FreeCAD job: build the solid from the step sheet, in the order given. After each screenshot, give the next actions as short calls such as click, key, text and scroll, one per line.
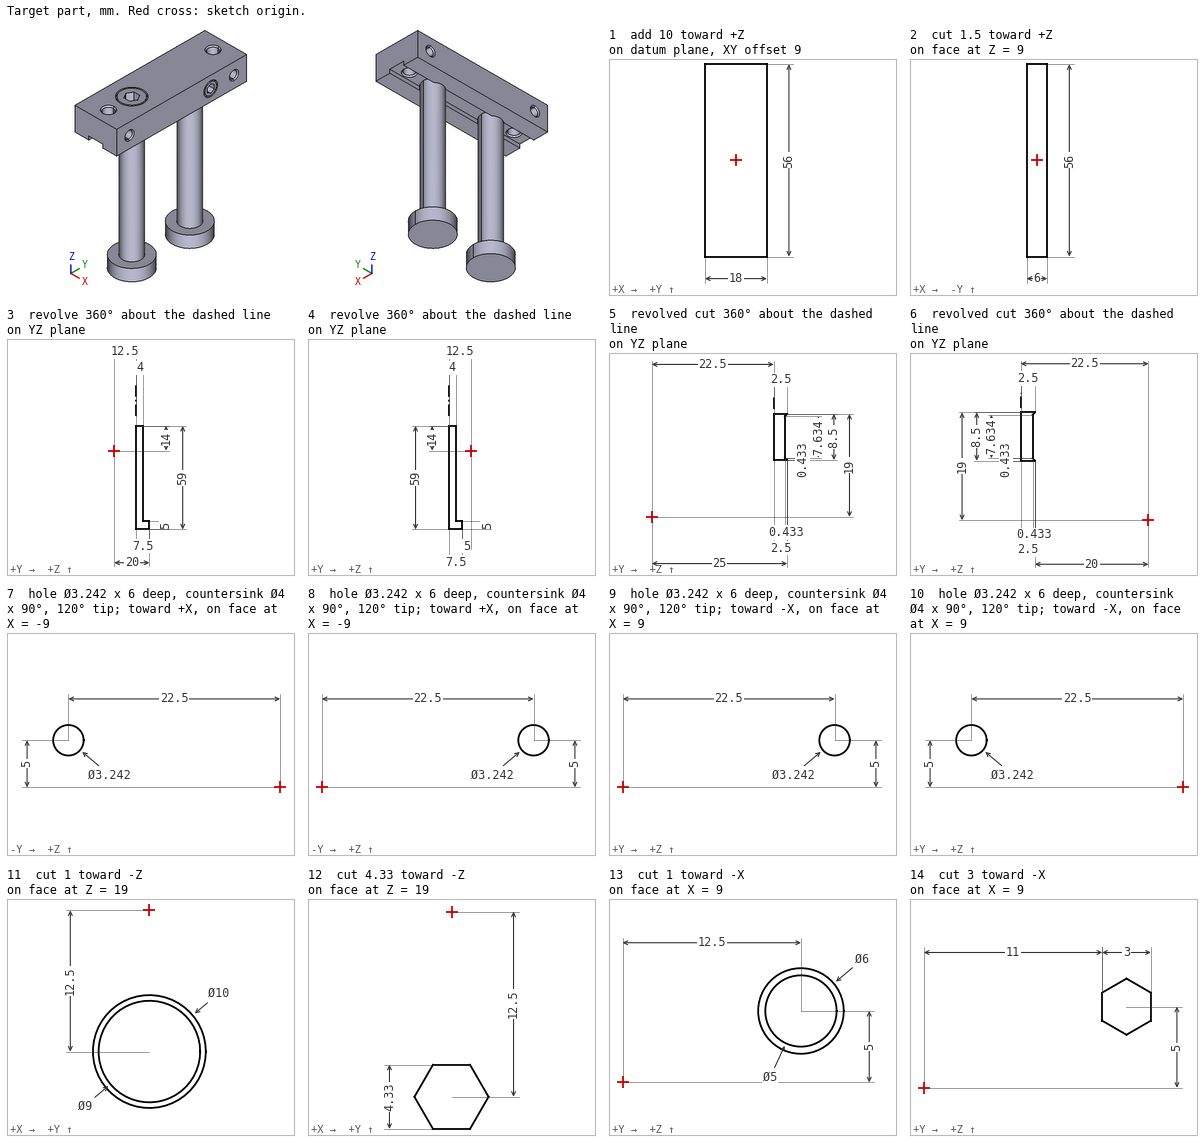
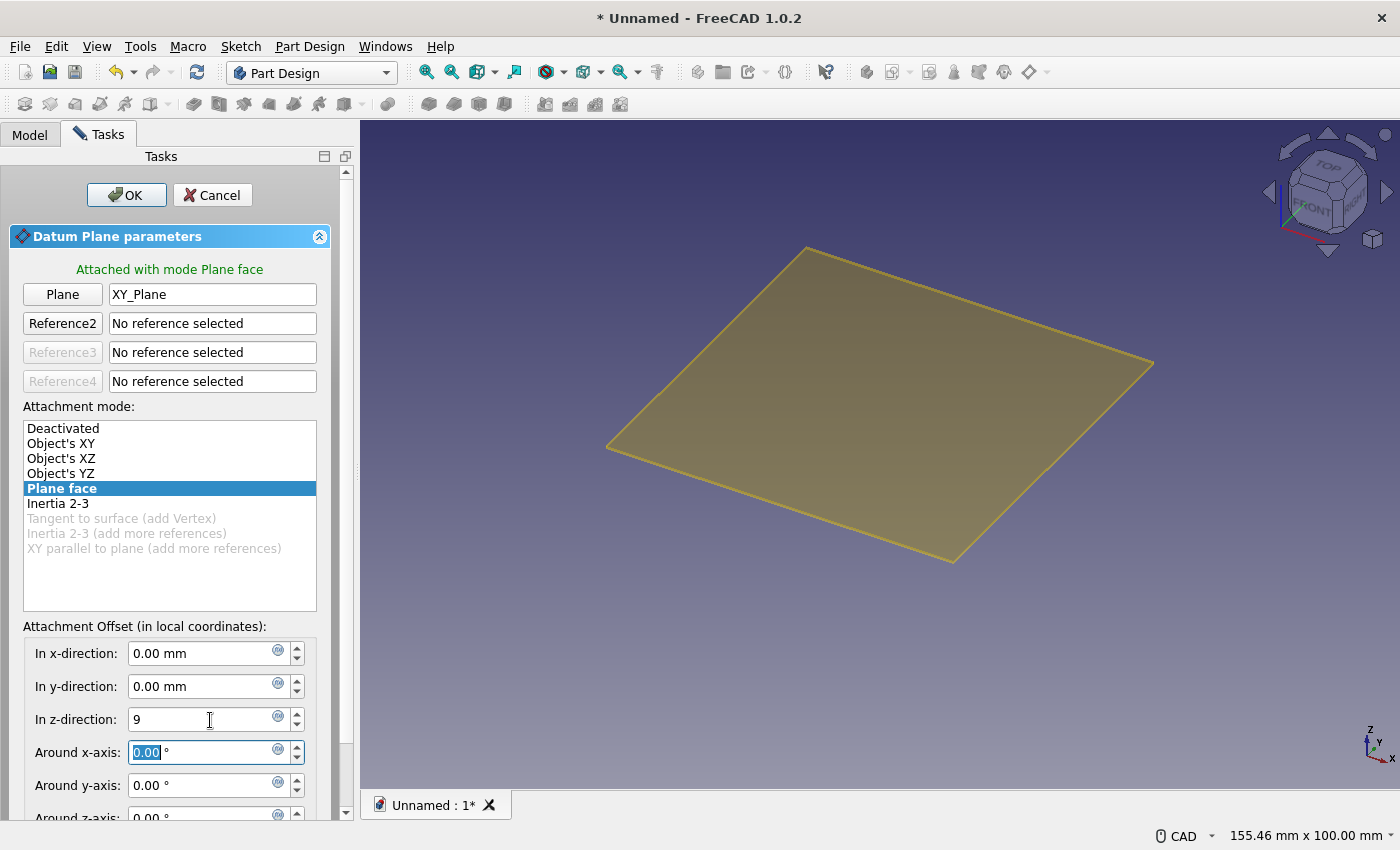
click(127, 195)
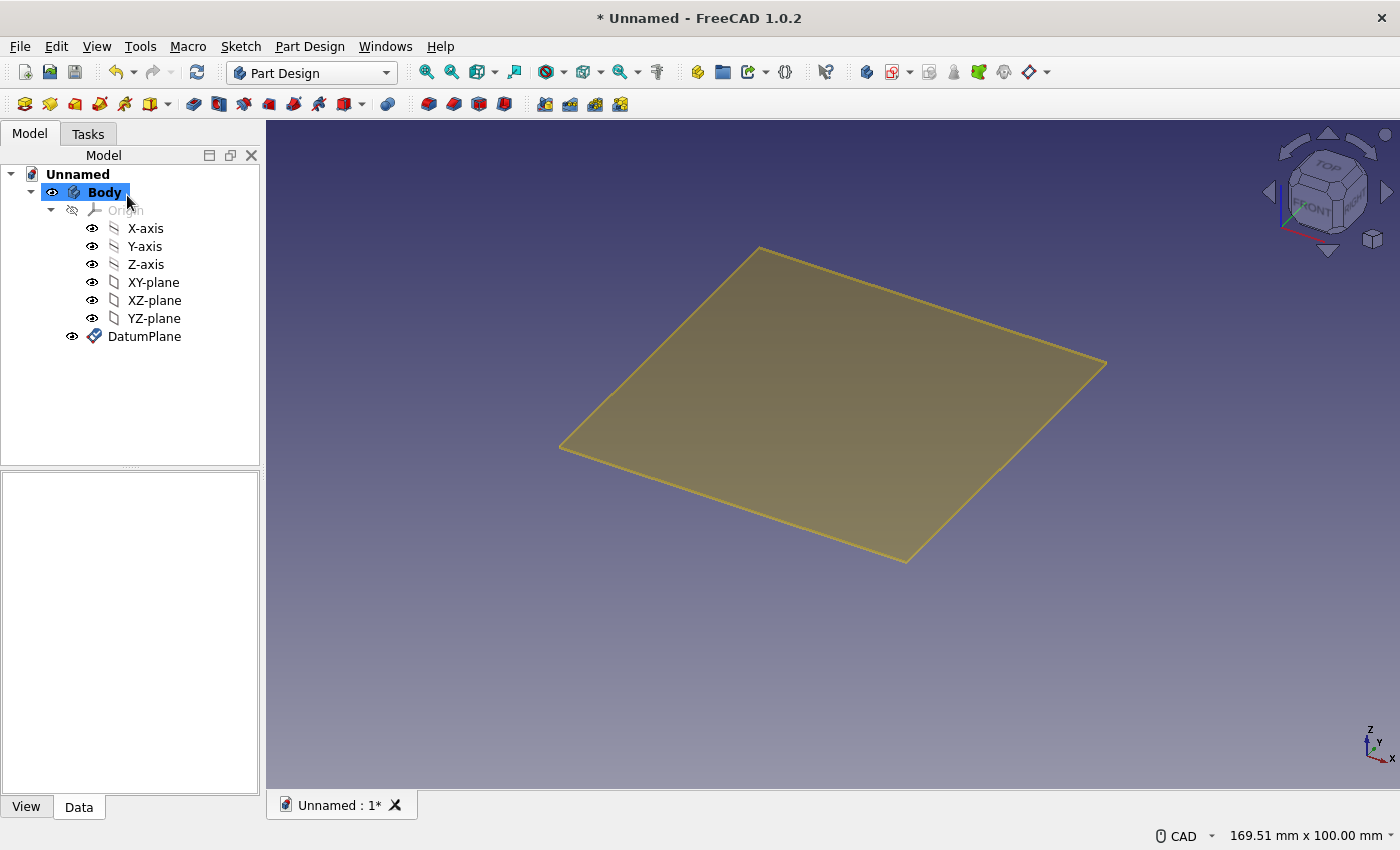
click(117, 336)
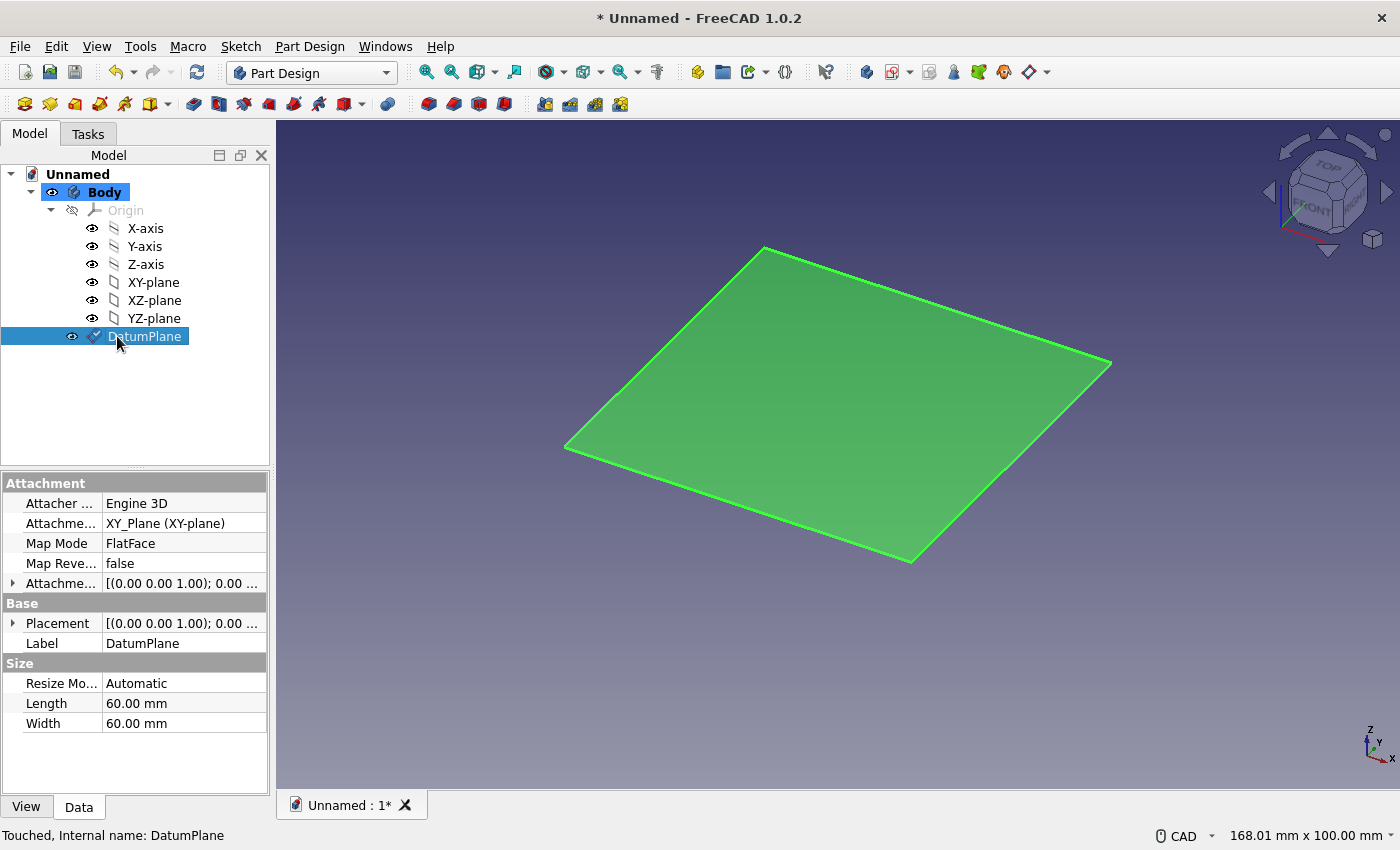
click(892, 72)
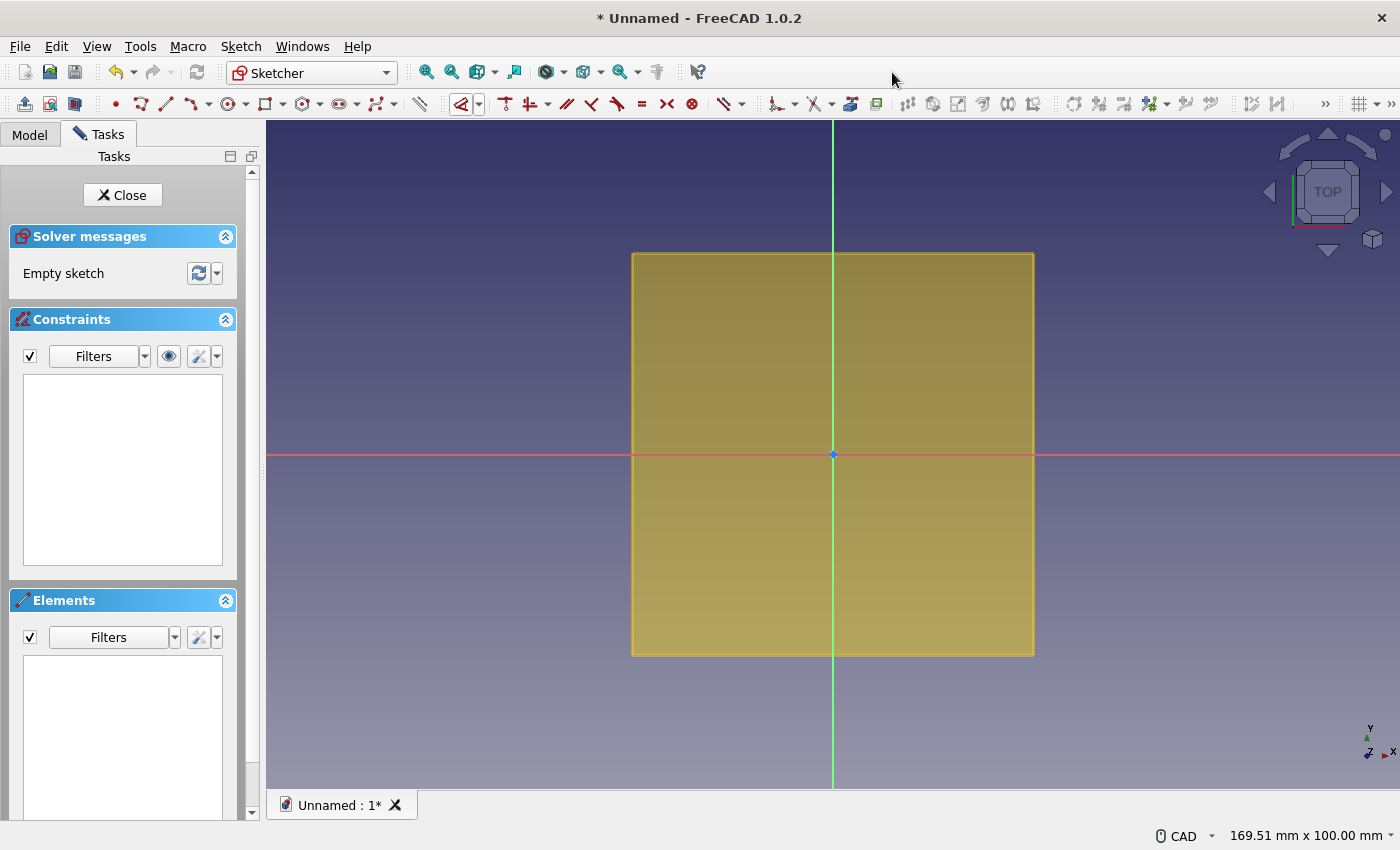
click(282, 104)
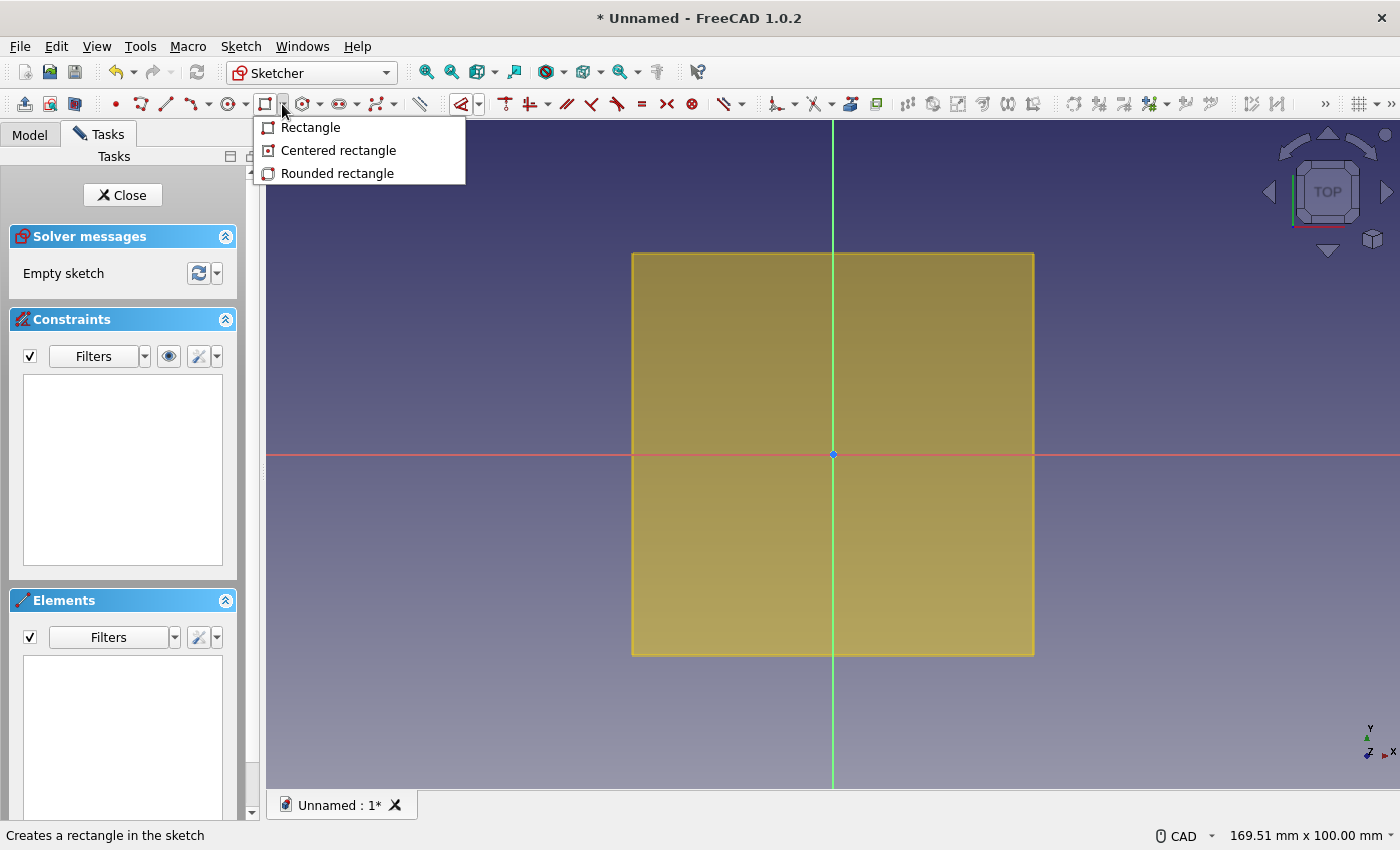
click(360, 150)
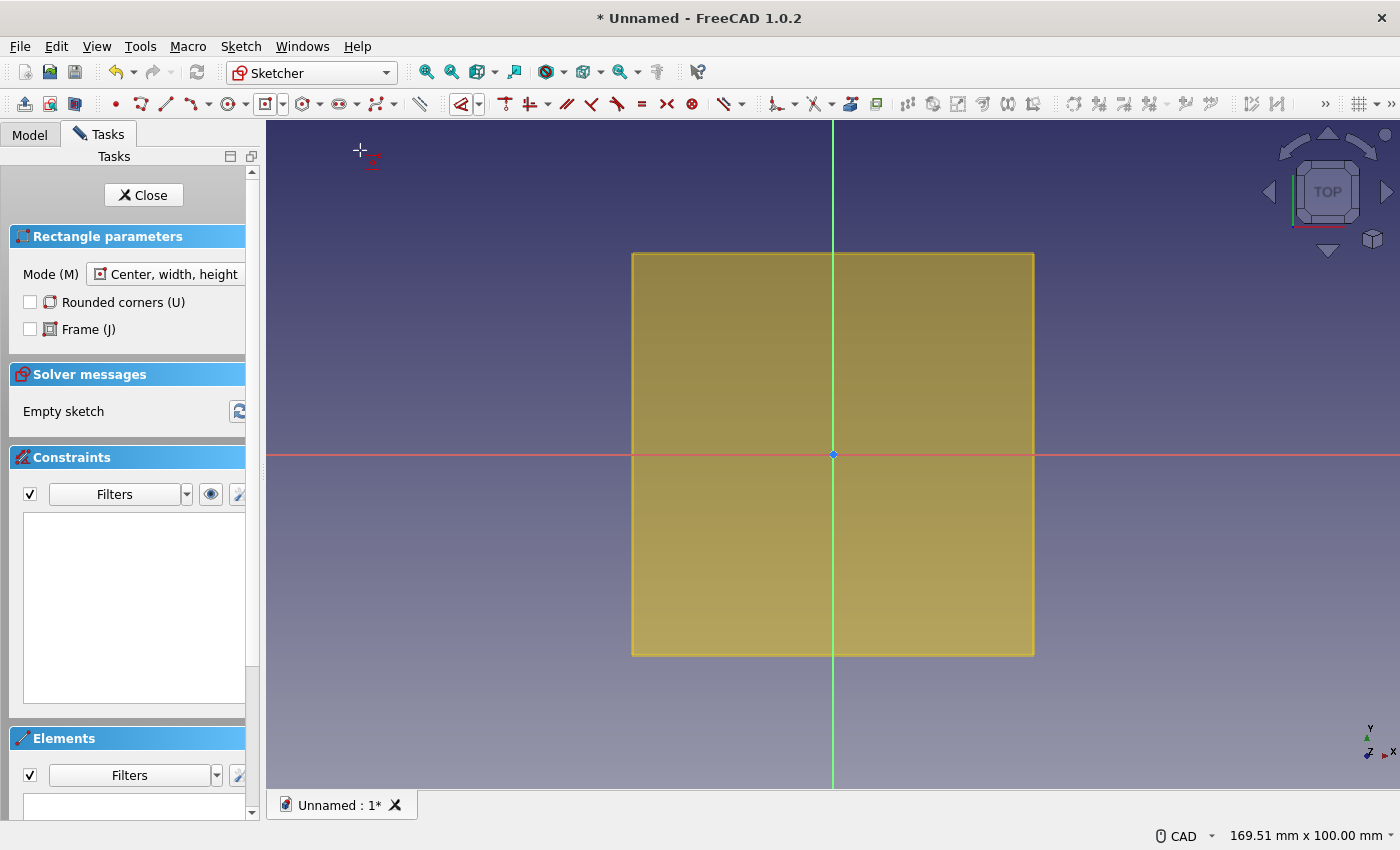
click(833, 454)
move(893, 267)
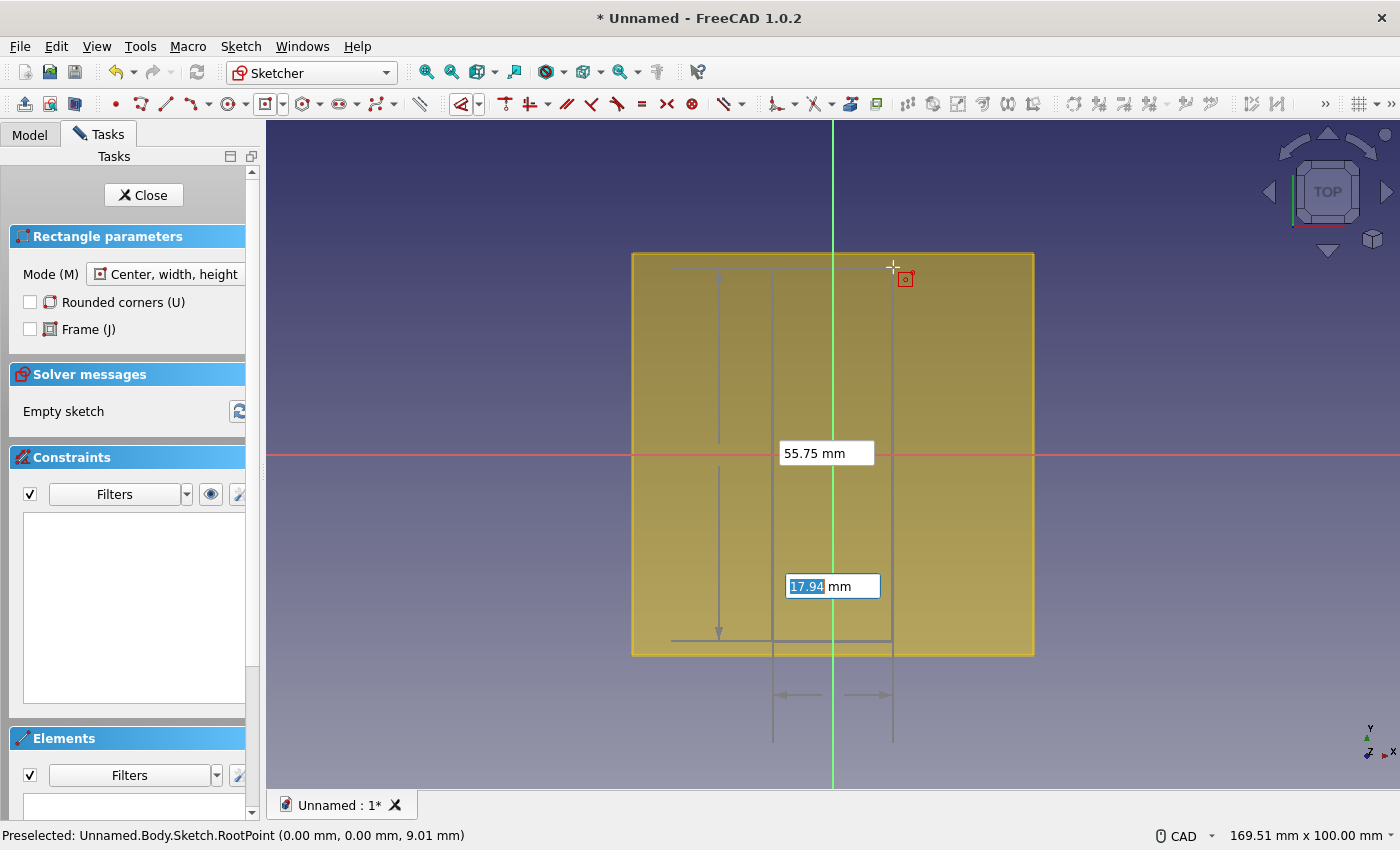
text(18)
key(Tab)
text(56)
key(Return)
key(Escape)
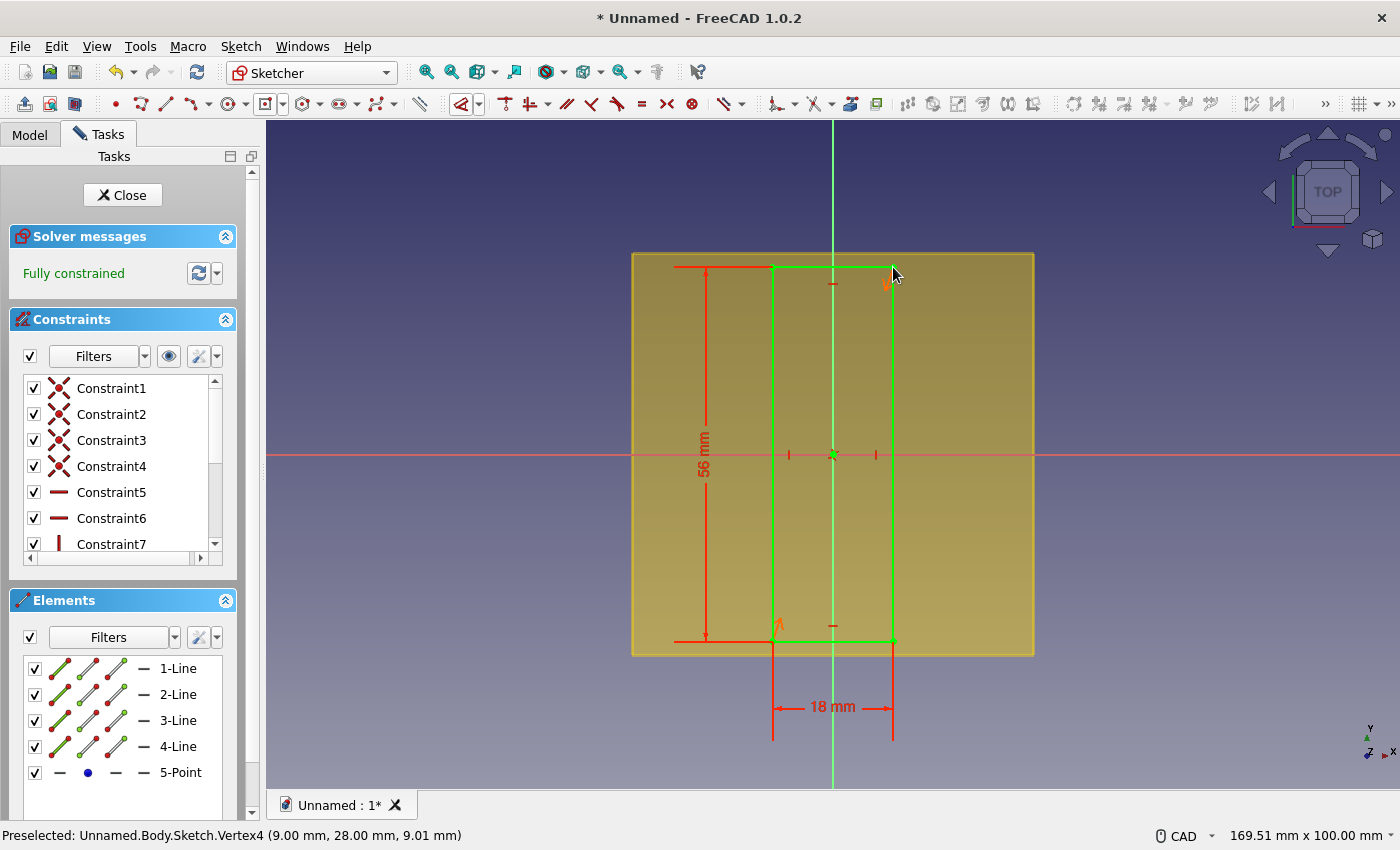
click(123, 195)